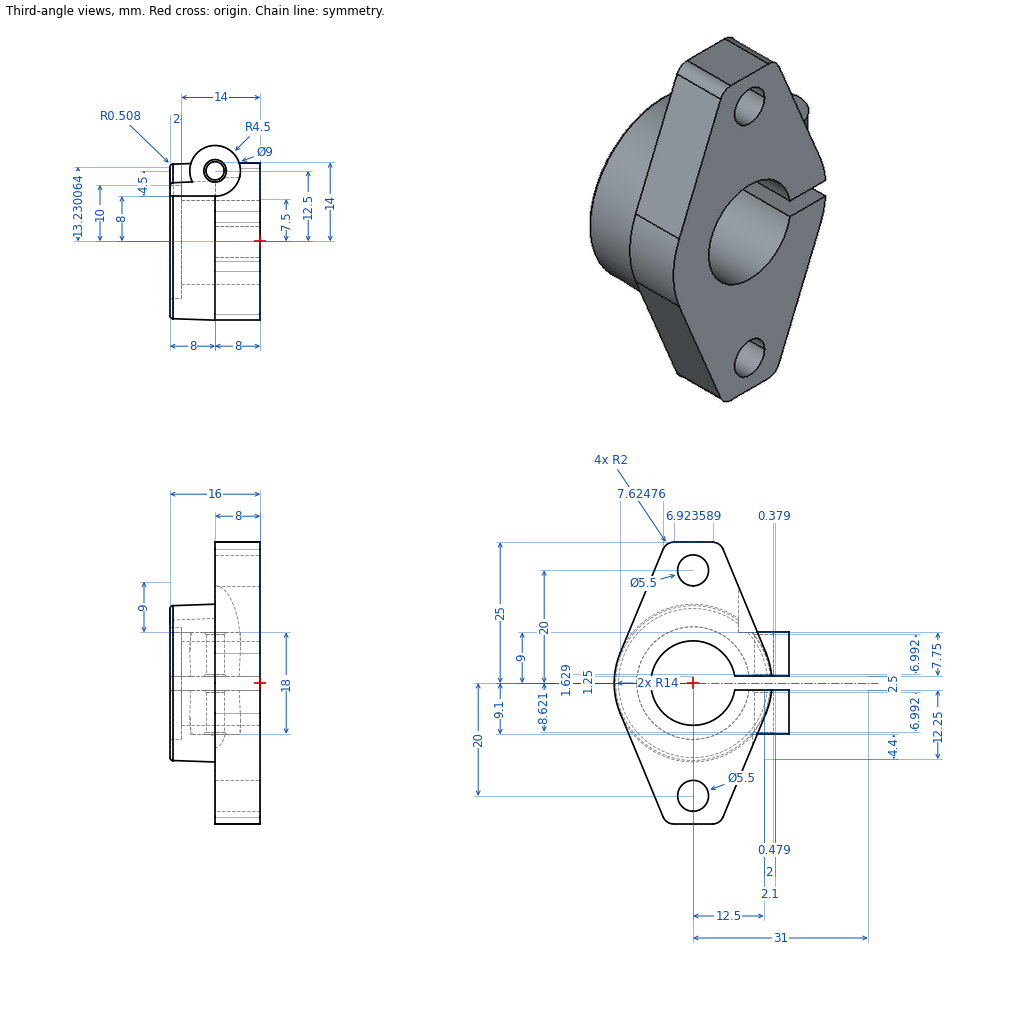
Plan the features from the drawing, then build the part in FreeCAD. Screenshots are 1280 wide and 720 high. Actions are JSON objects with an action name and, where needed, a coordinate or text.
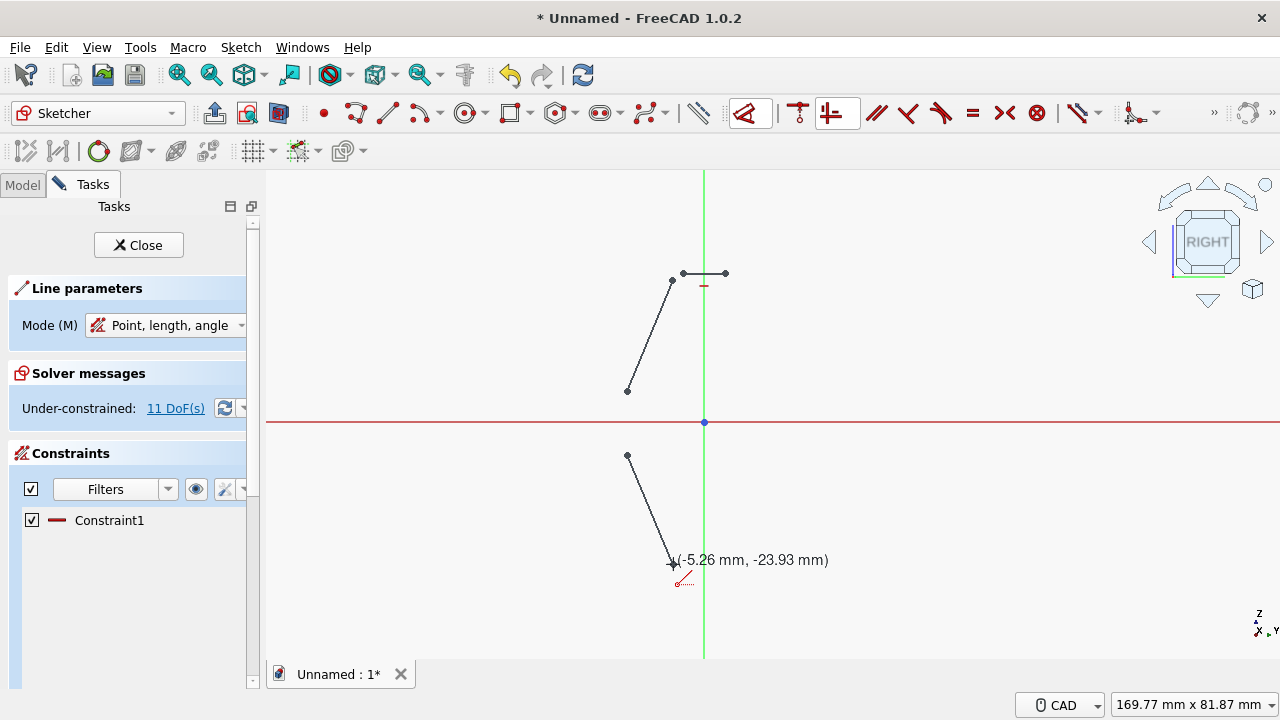
{"action": "left_click", "coordinate": [684, 571]}
{"action": "left_click", "coordinate": [725, 571]}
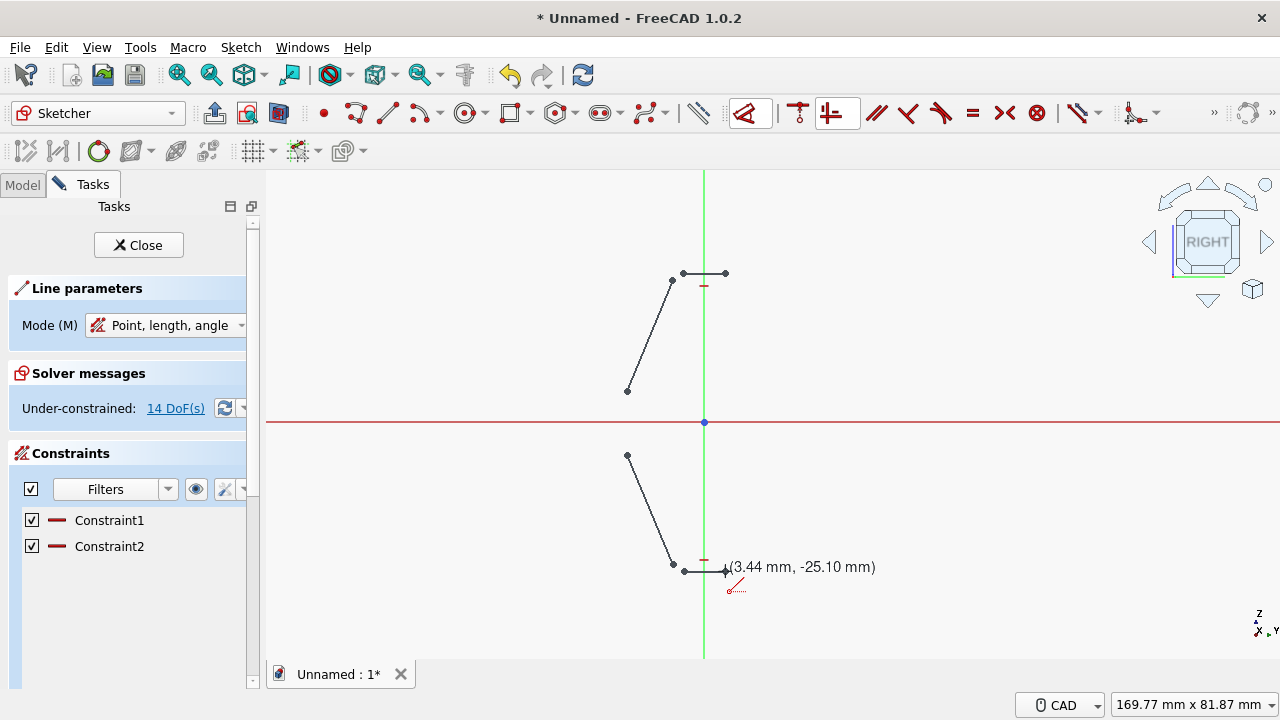
{"action": "left_click", "coordinate": [736, 564]}
{"action": "left_click", "coordinate": [782, 454]}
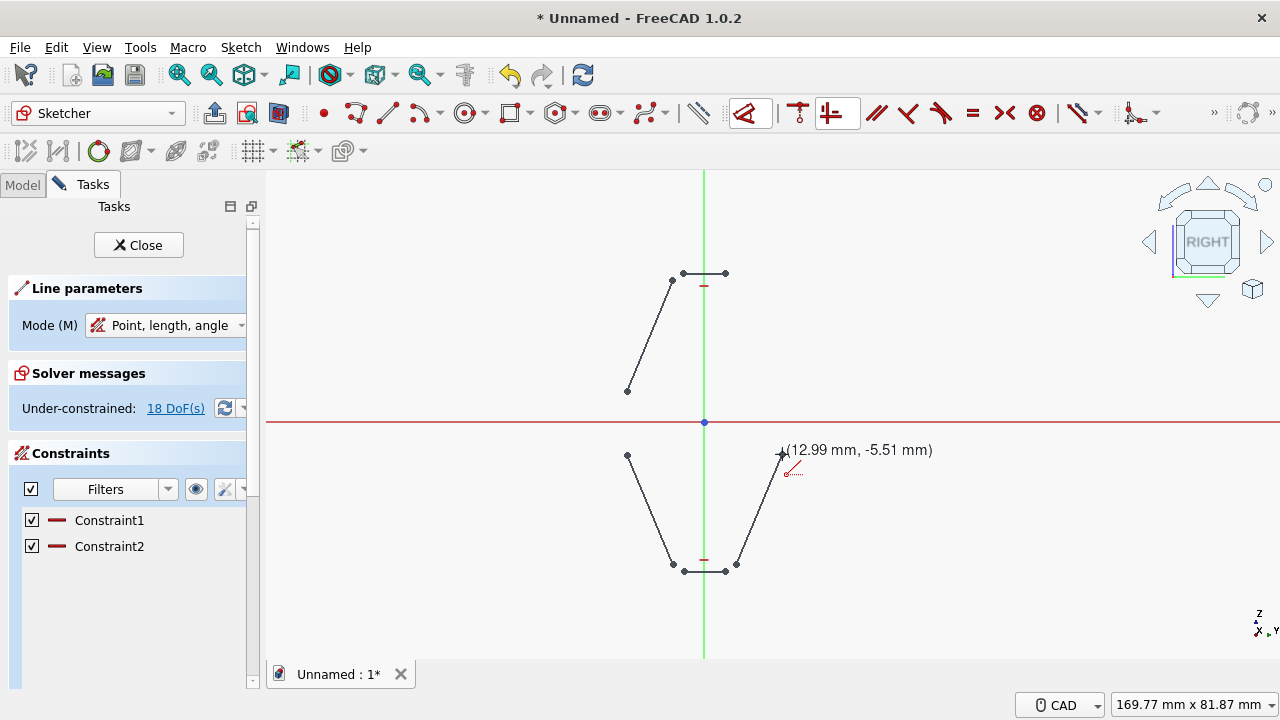
{"action": "left_click", "coordinate": [782, 390]}
{"action": "left_click", "coordinate": [736, 280]}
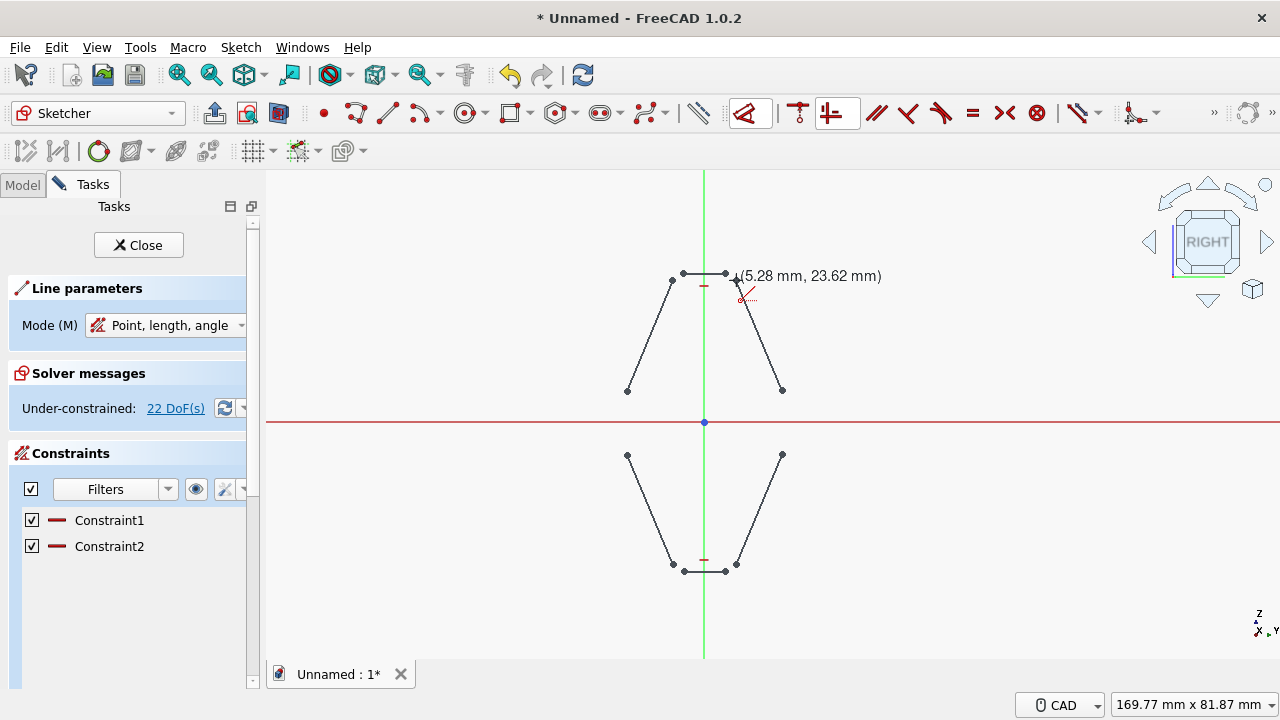
{"action": "key", "text": "g 3 a"}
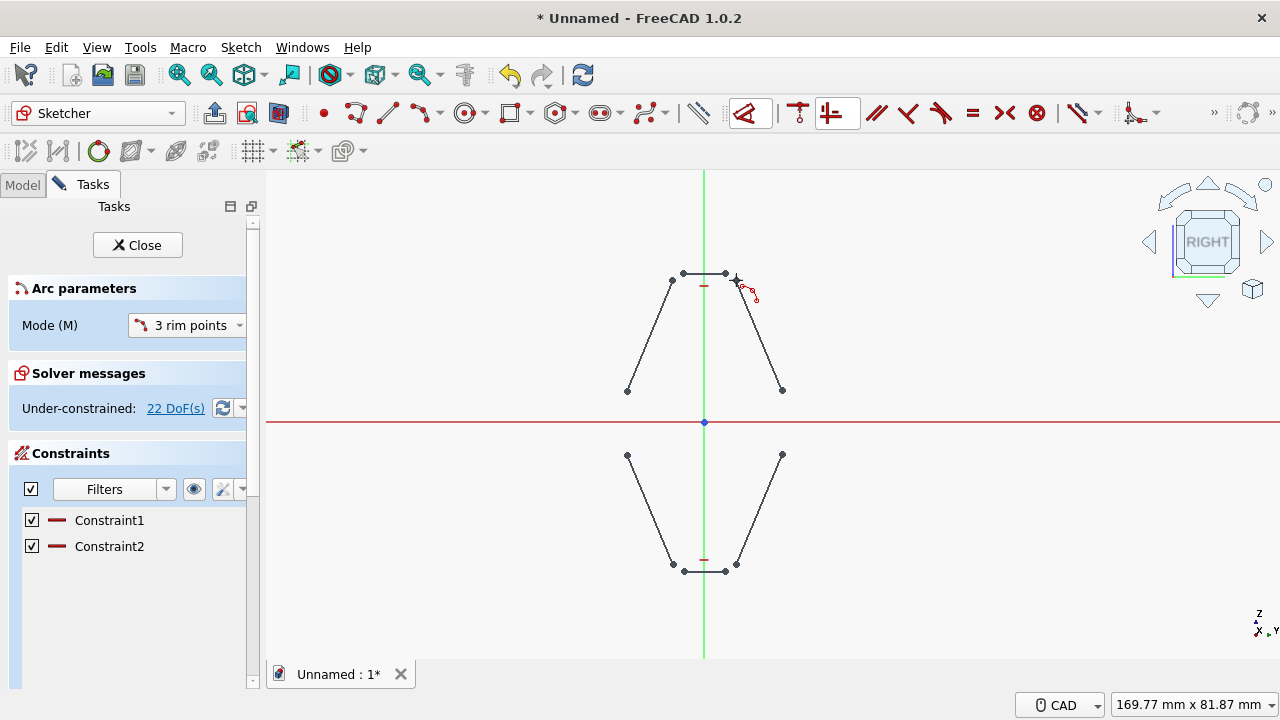
{"action": "left_click", "coordinate": [684, 274]}
{"action": "left_click", "coordinate": [673, 281]}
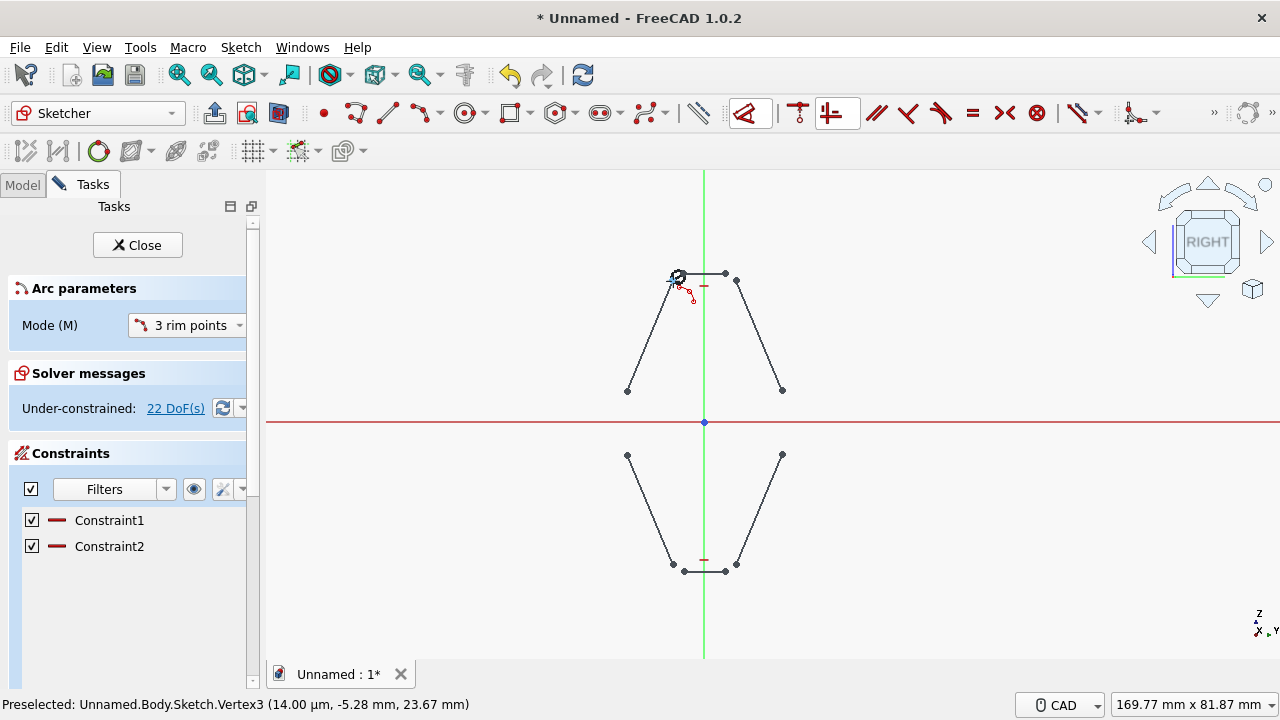
{"action": "scroll", "coordinate": [677, 275], "scroll_direction": "up", "scroll_amount": 11}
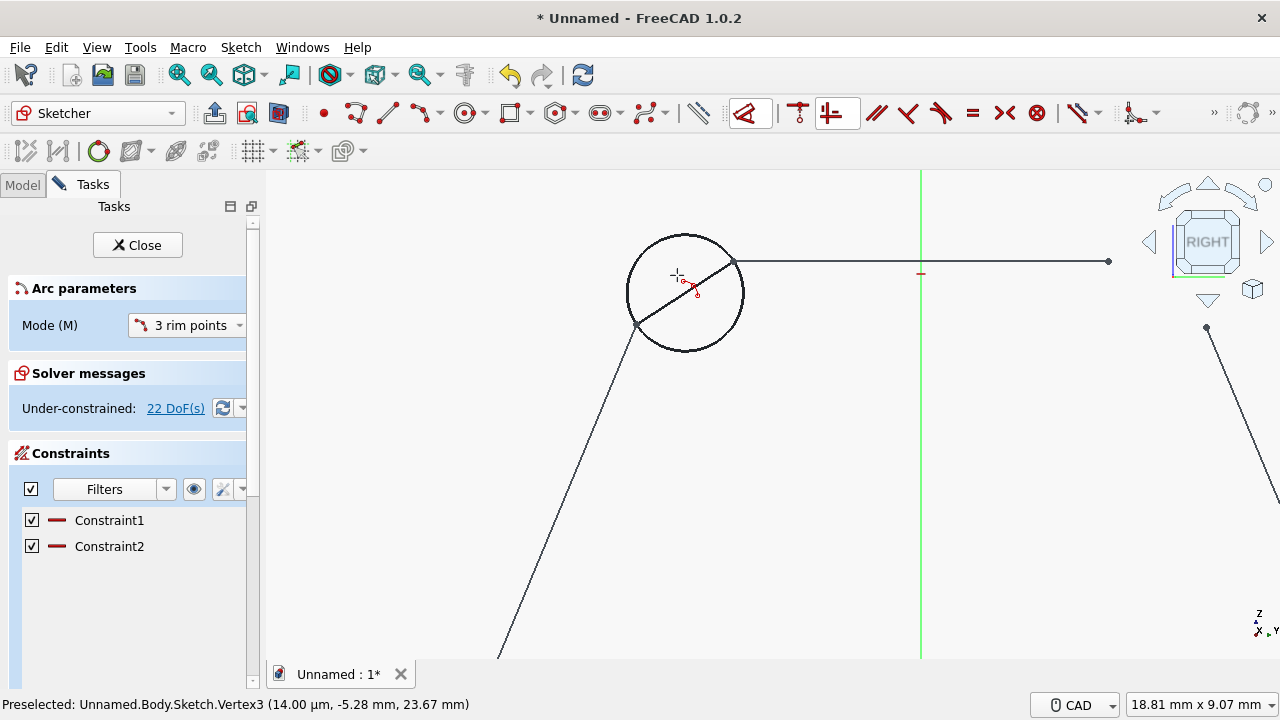
{"action": "left_click", "coordinate": [675, 271]}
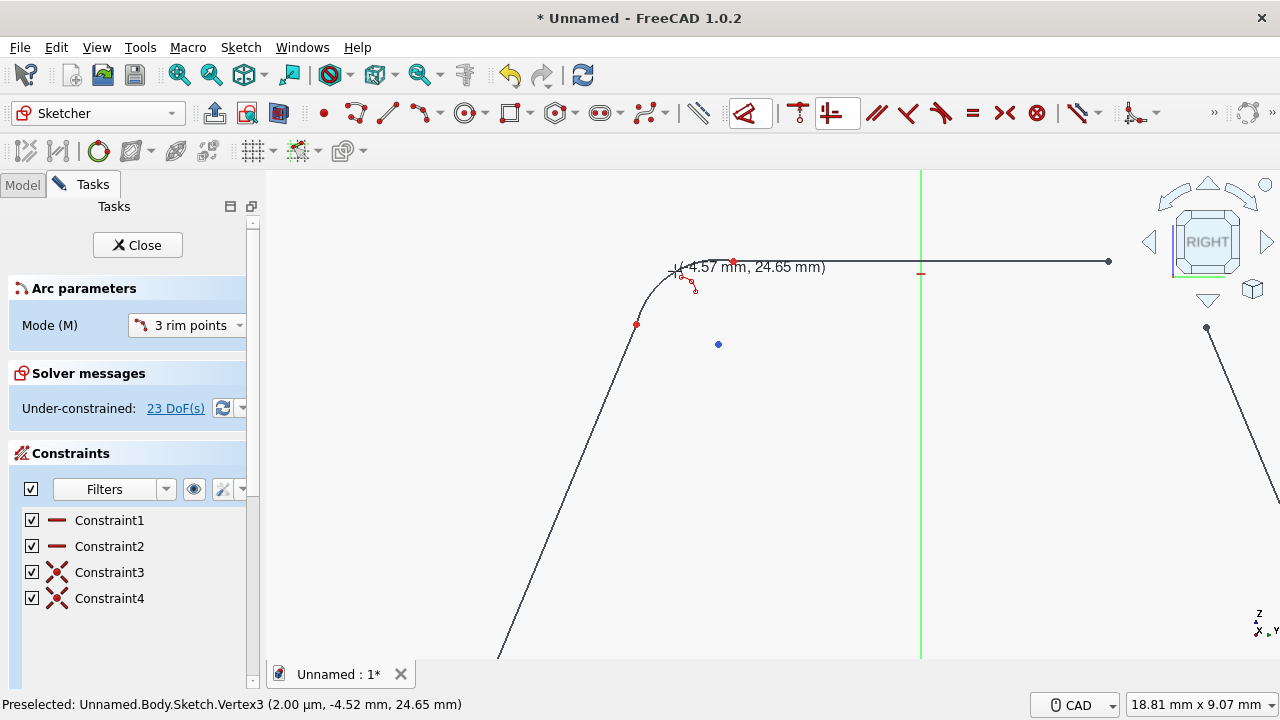
{"action": "scroll", "coordinate": [677, 267], "scroll_direction": "down", "scroll_amount": 11}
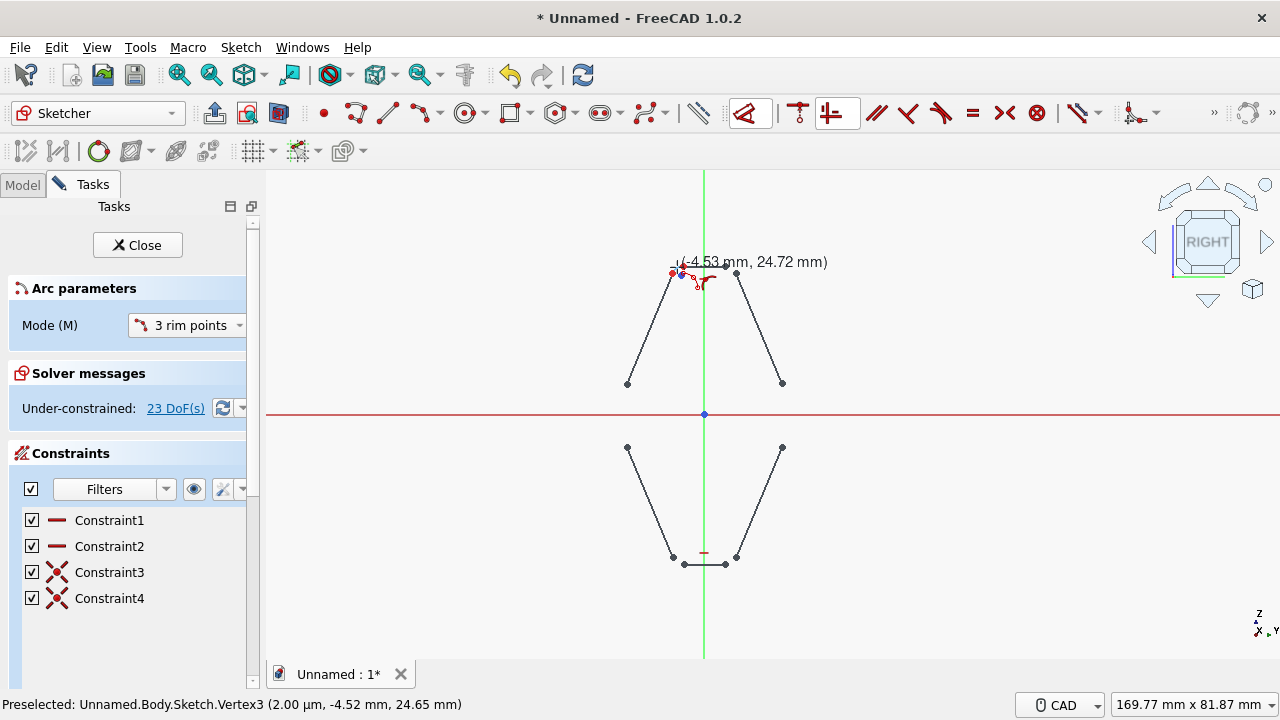
{"action": "left_click", "coordinate": [627, 384]}
{"action": "left_click", "coordinate": [627, 448]}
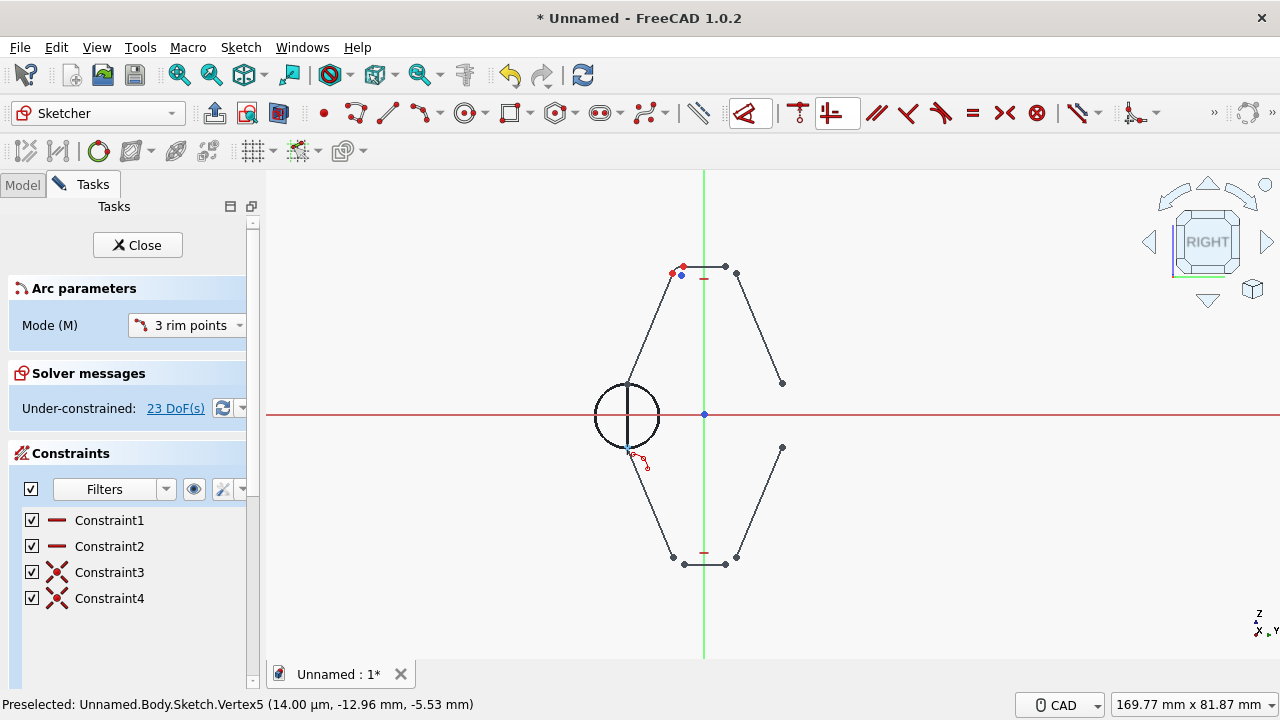
{"action": "scroll", "coordinate": [621, 408], "scroll_direction": "up", "scroll_amount": 5}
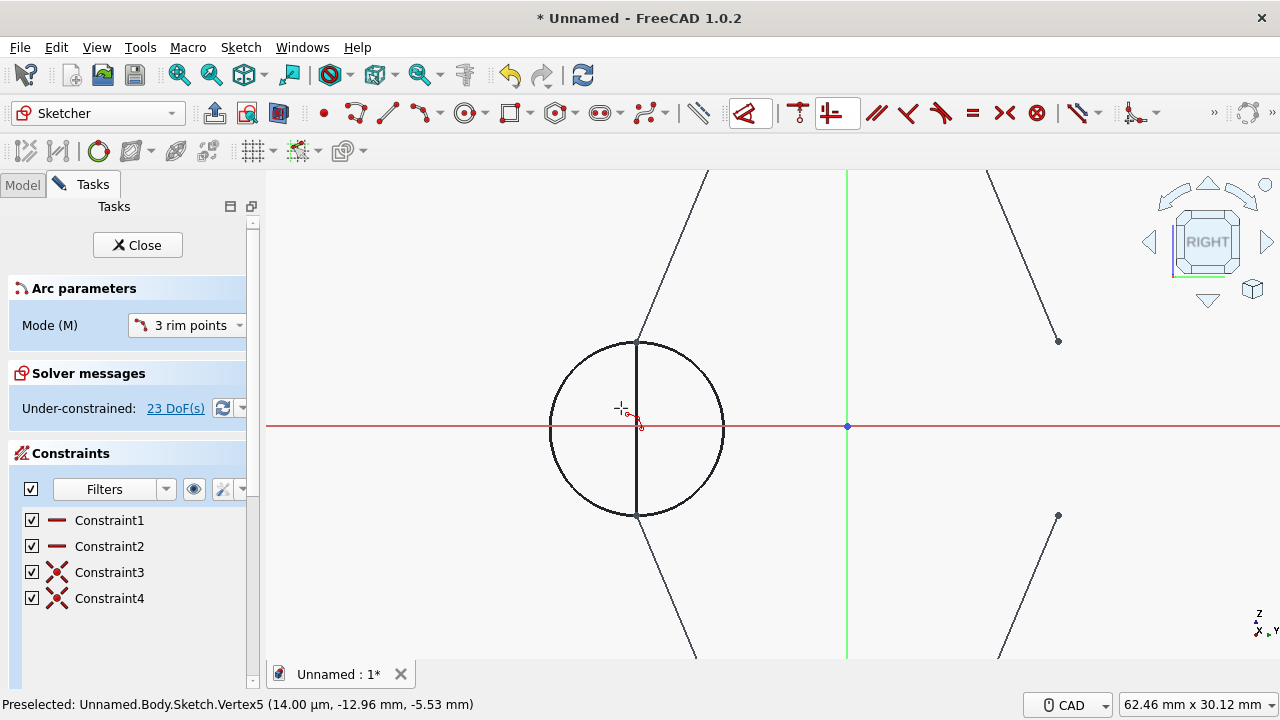
{"action": "left_click", "coordinate": [621, 408]}